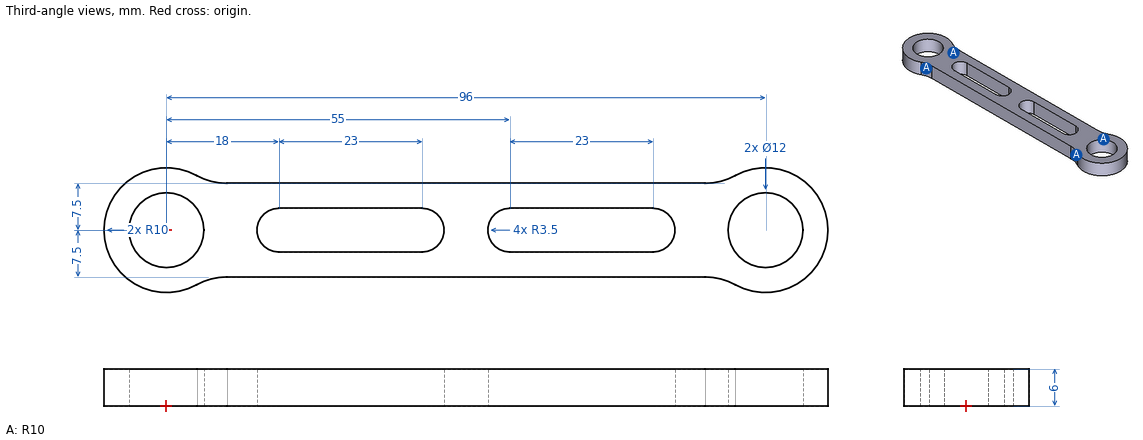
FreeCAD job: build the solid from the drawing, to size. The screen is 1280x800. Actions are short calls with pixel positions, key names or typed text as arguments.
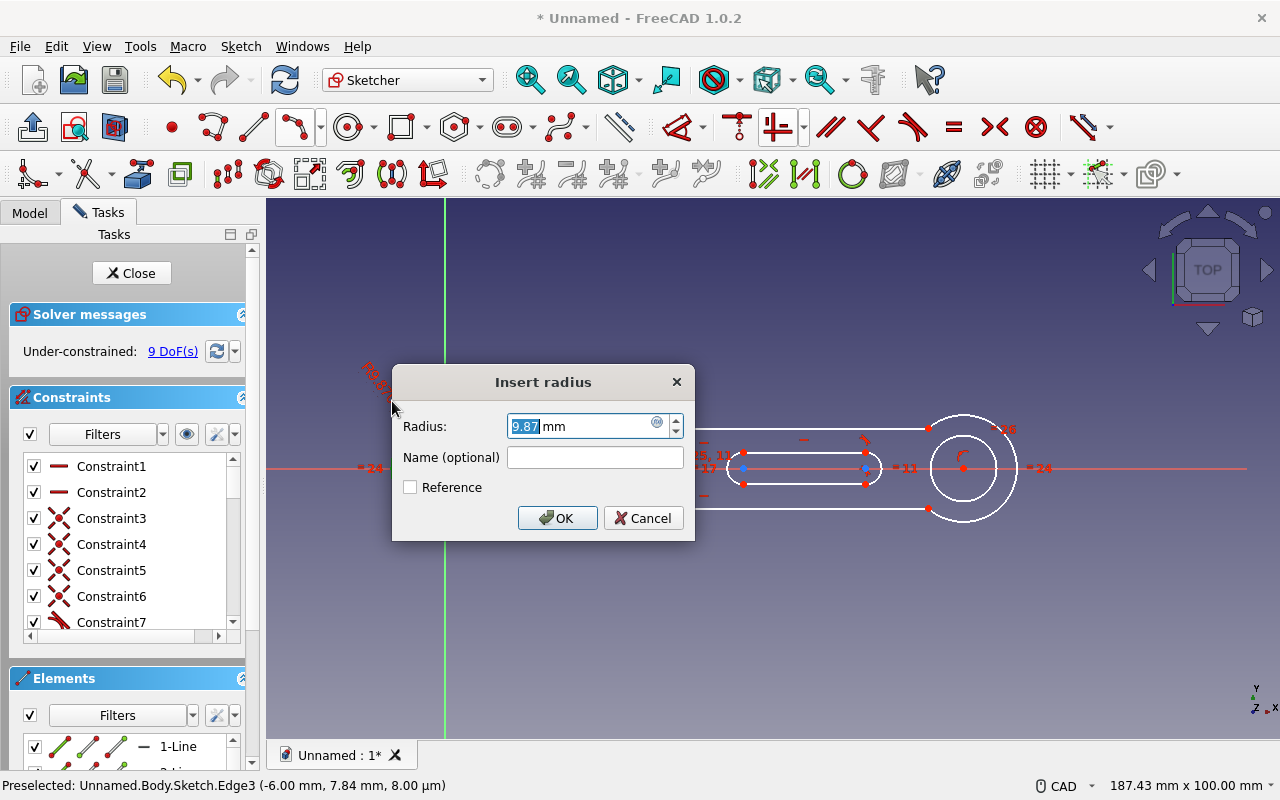
text(10)
key(Return)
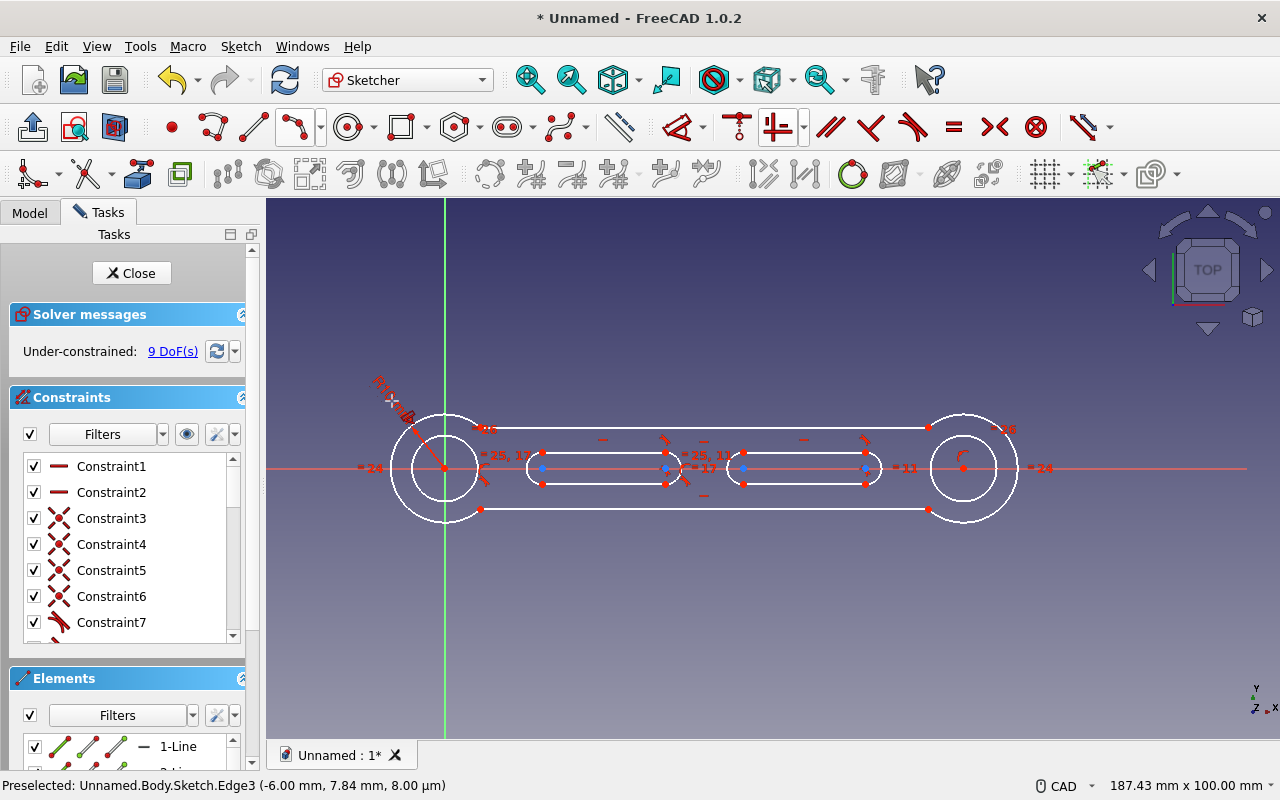
scroll(730, 459, up, 4)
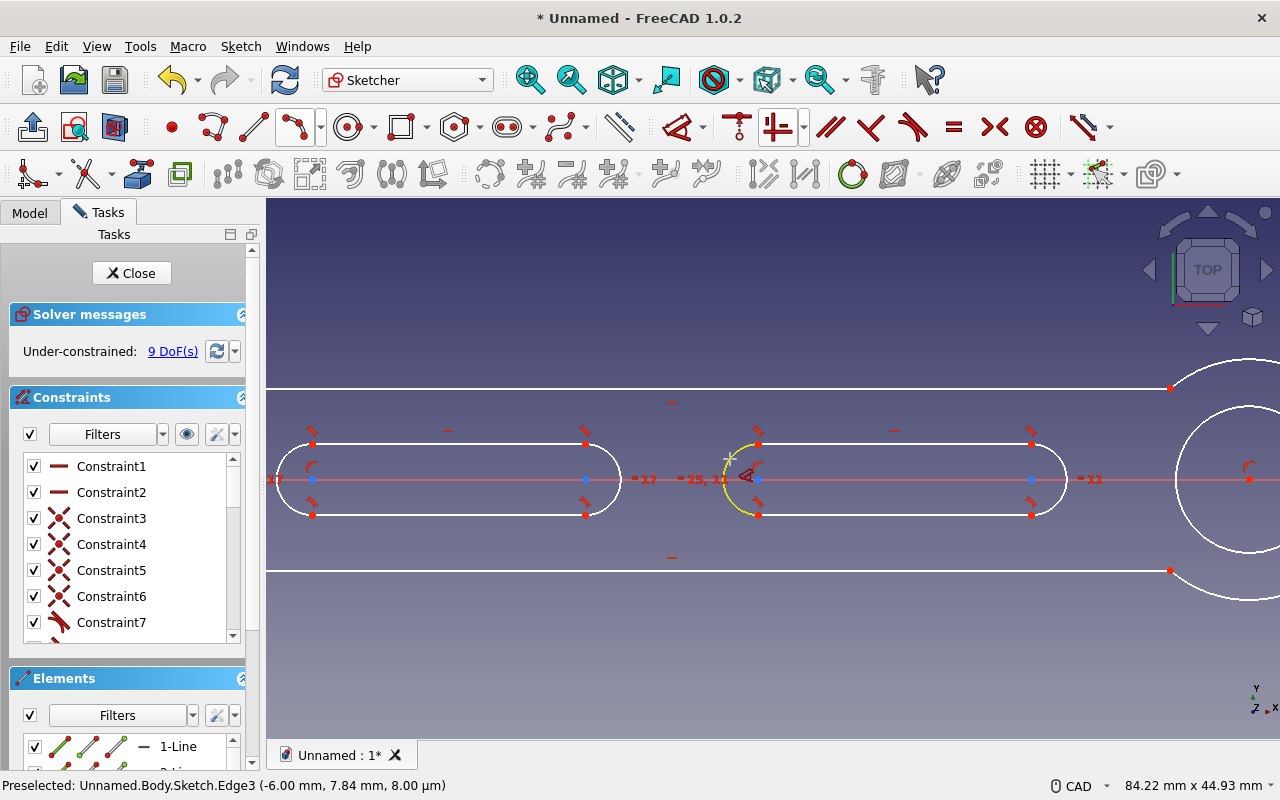
click(730, 459)
click(704, 440)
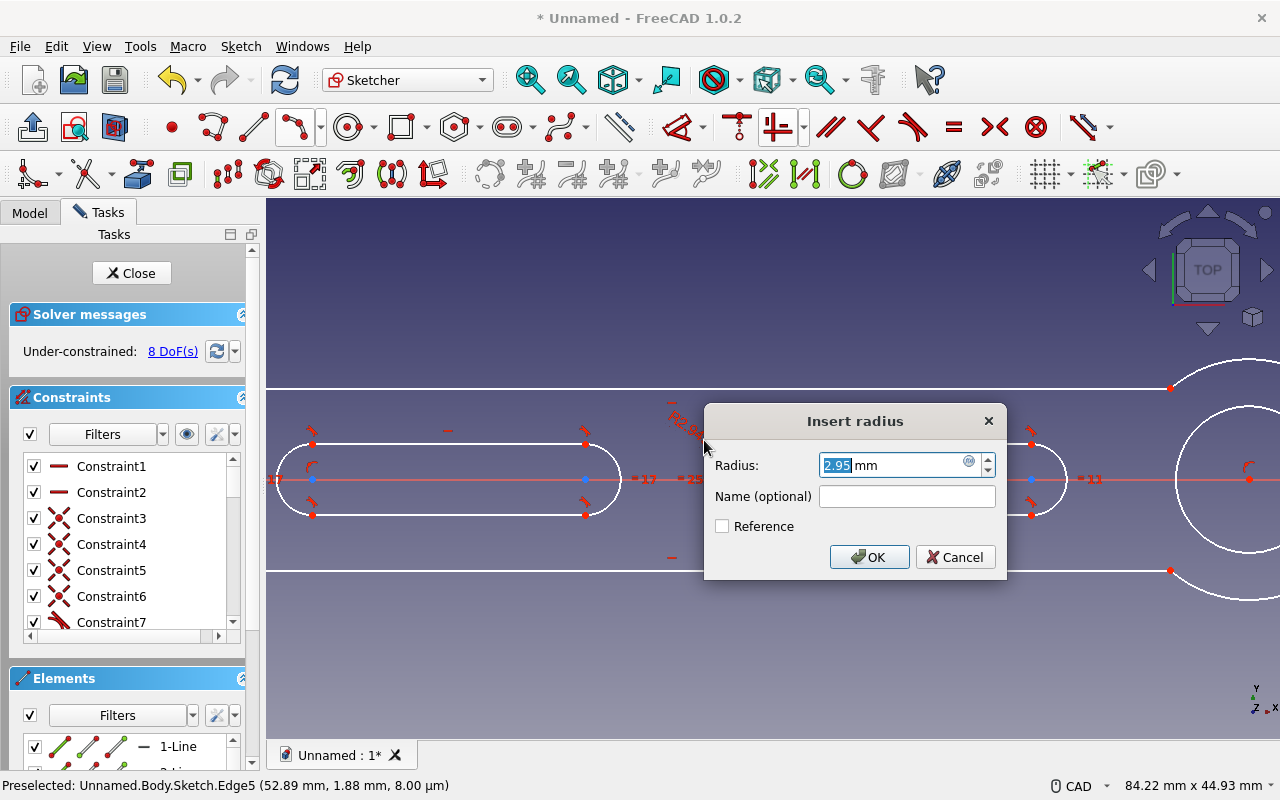
text(3.5)
key(Return)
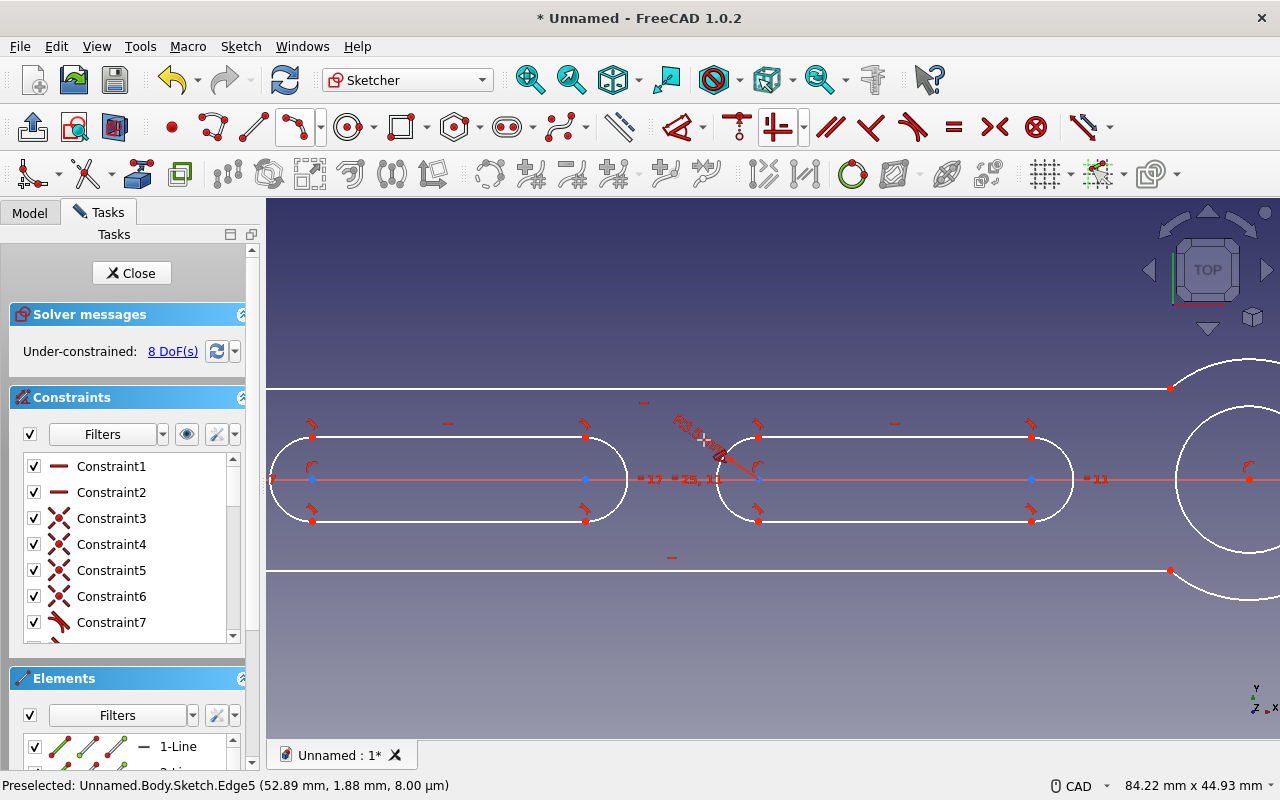
scroll(730, 459, down, 4)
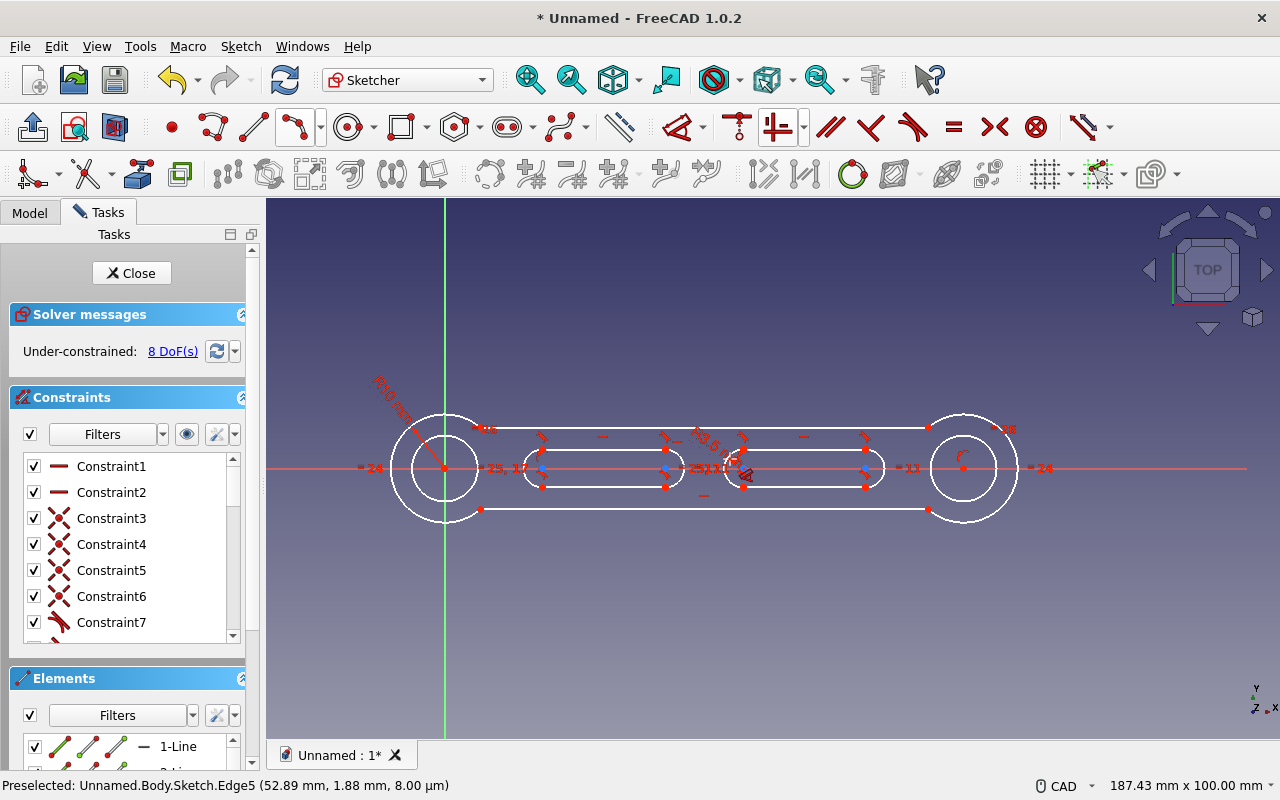
click(987, 445)
click(1026, 406)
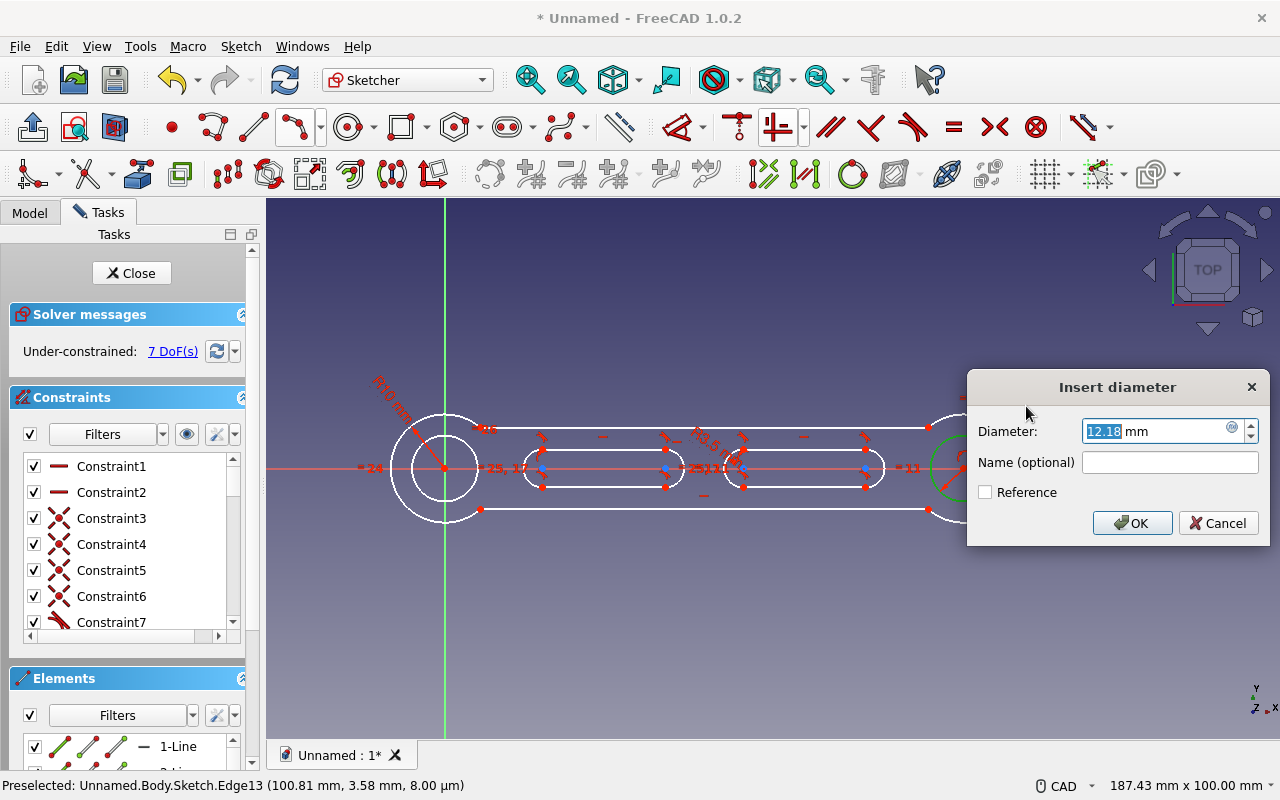
text(12)
key(Return)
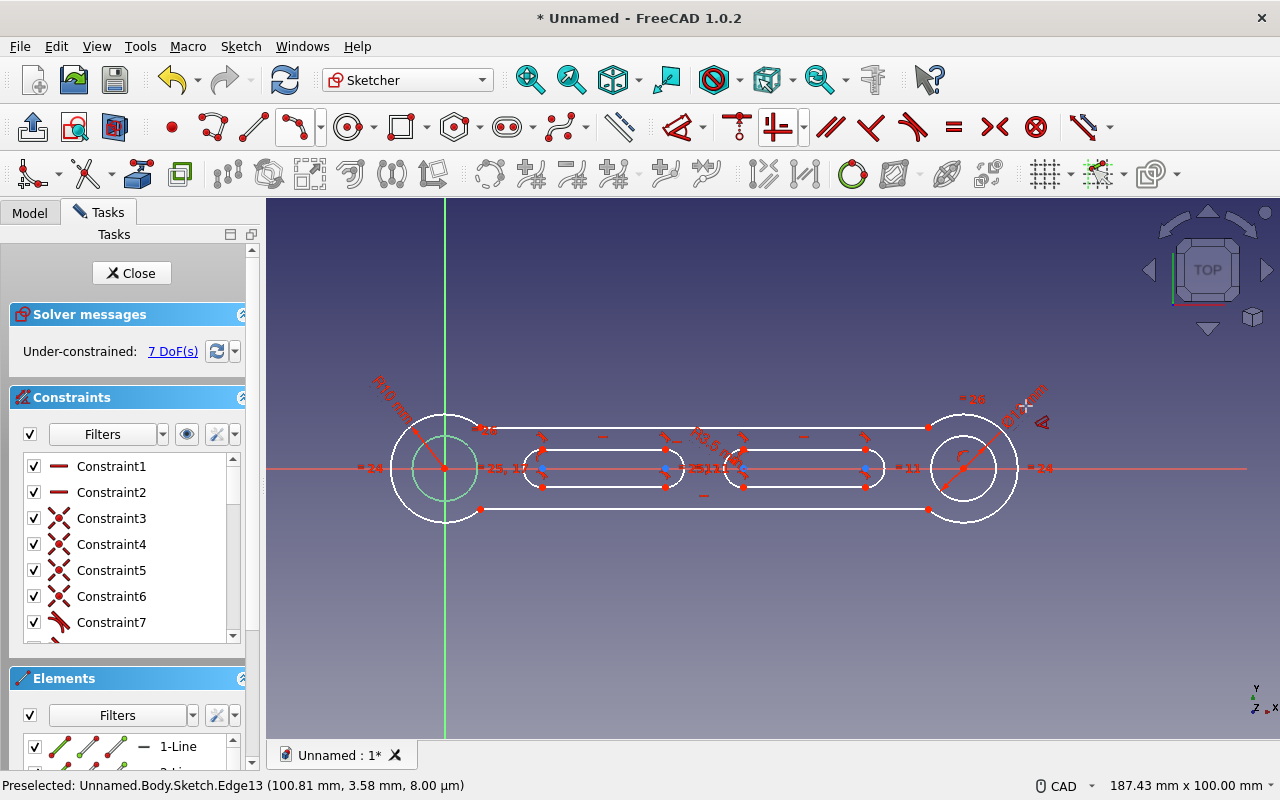
click(780, 450)
click(804, 392)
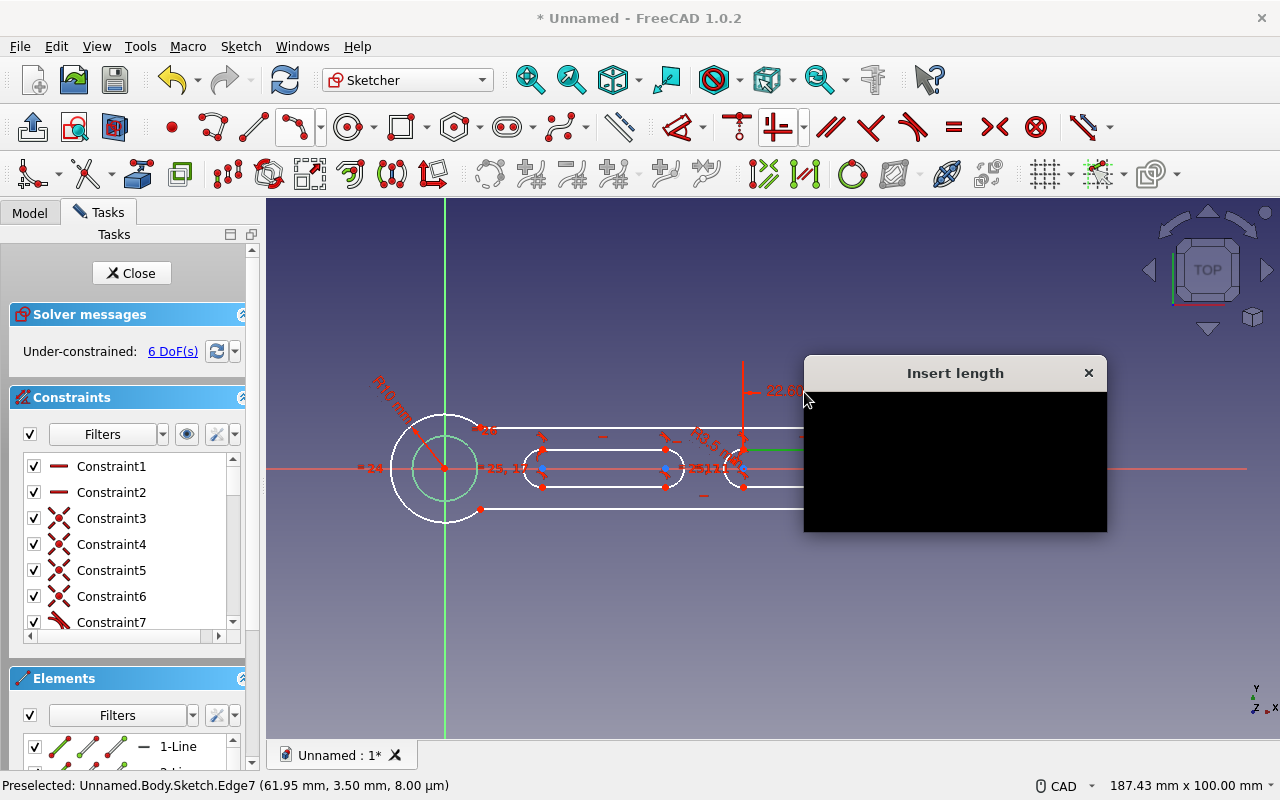
text(23)
key(Return)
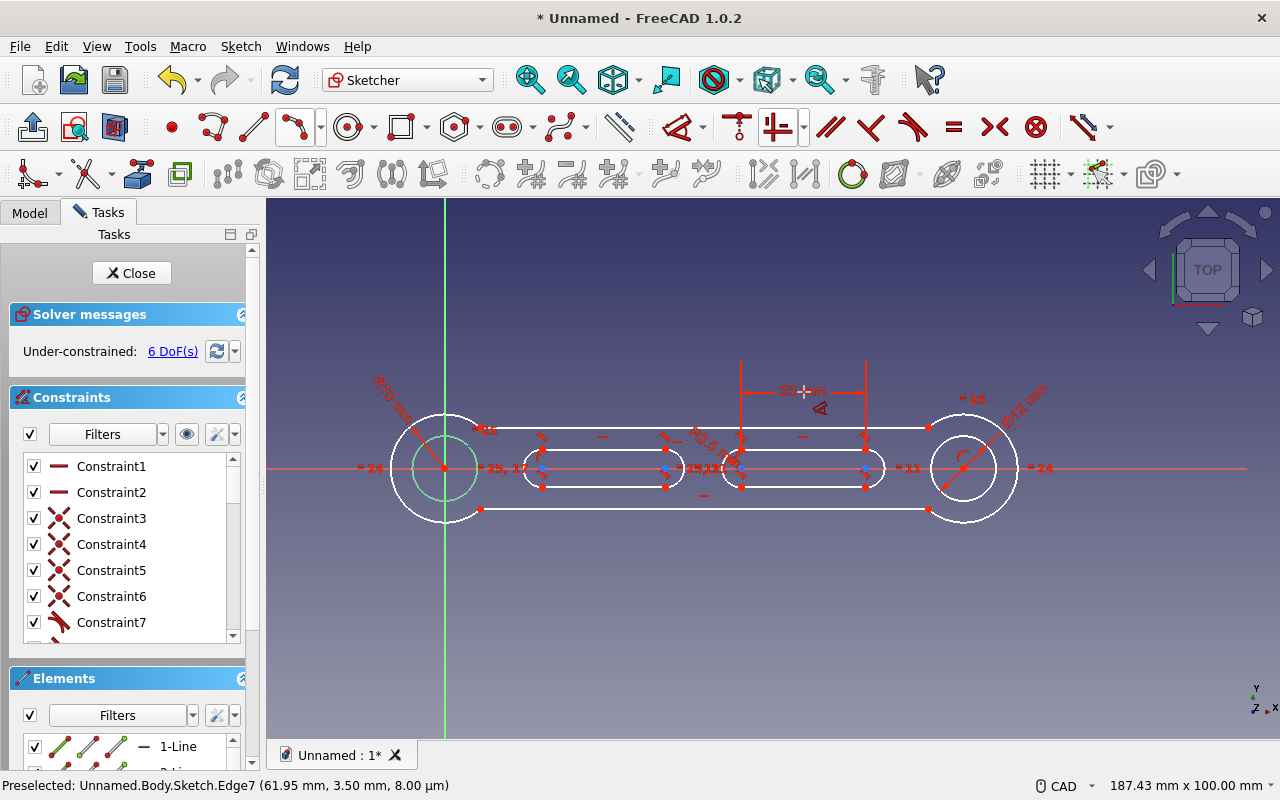
click(579, 450)
click(604, 392)